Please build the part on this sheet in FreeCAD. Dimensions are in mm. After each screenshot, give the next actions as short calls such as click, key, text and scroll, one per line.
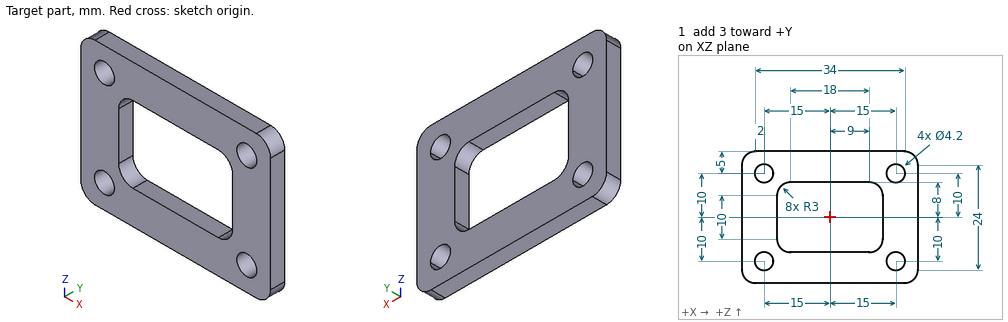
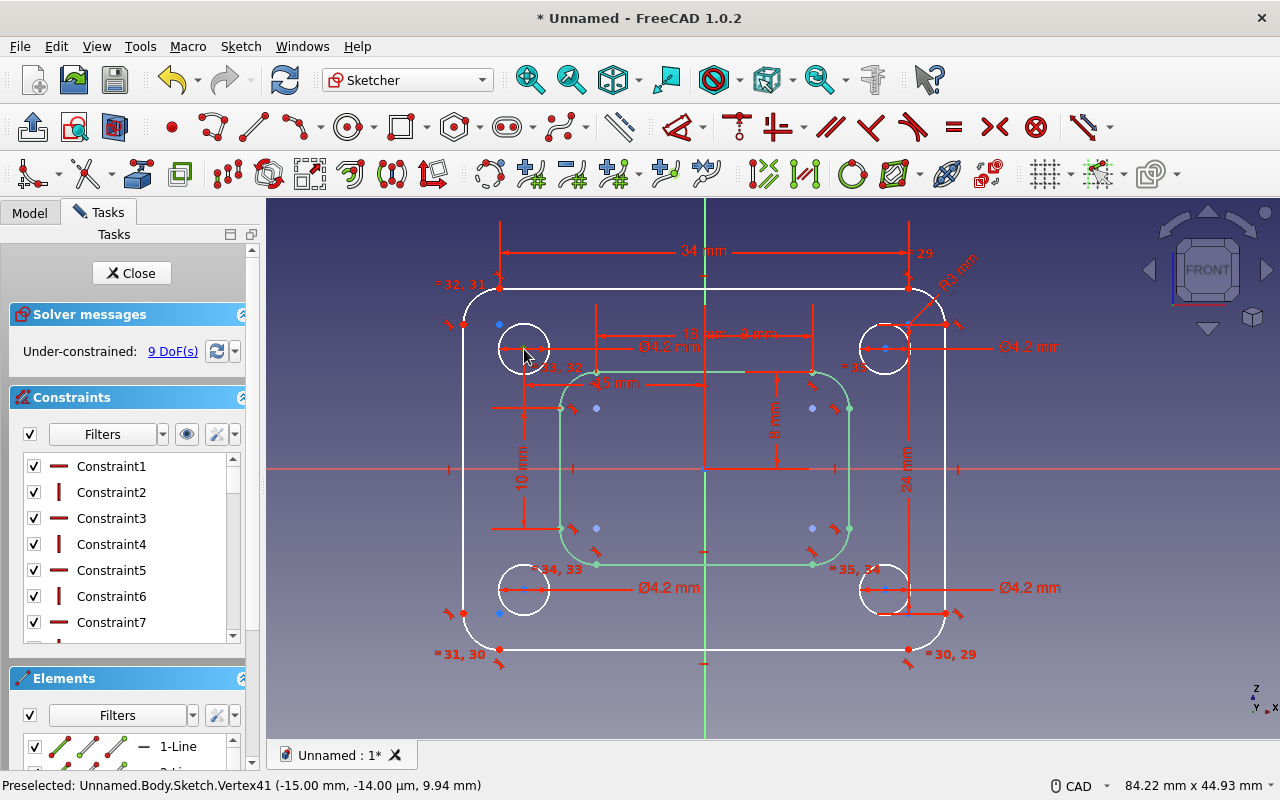
key(i)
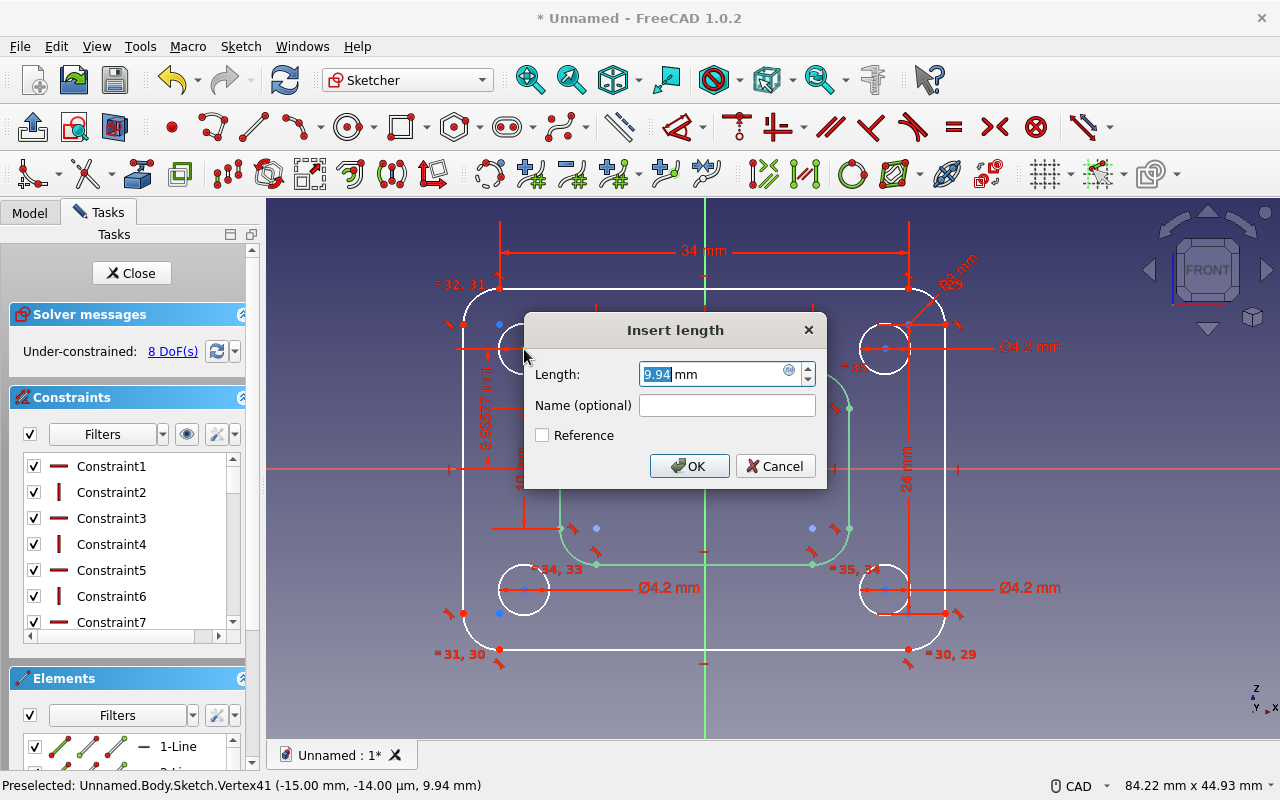
text(10)
key(Return)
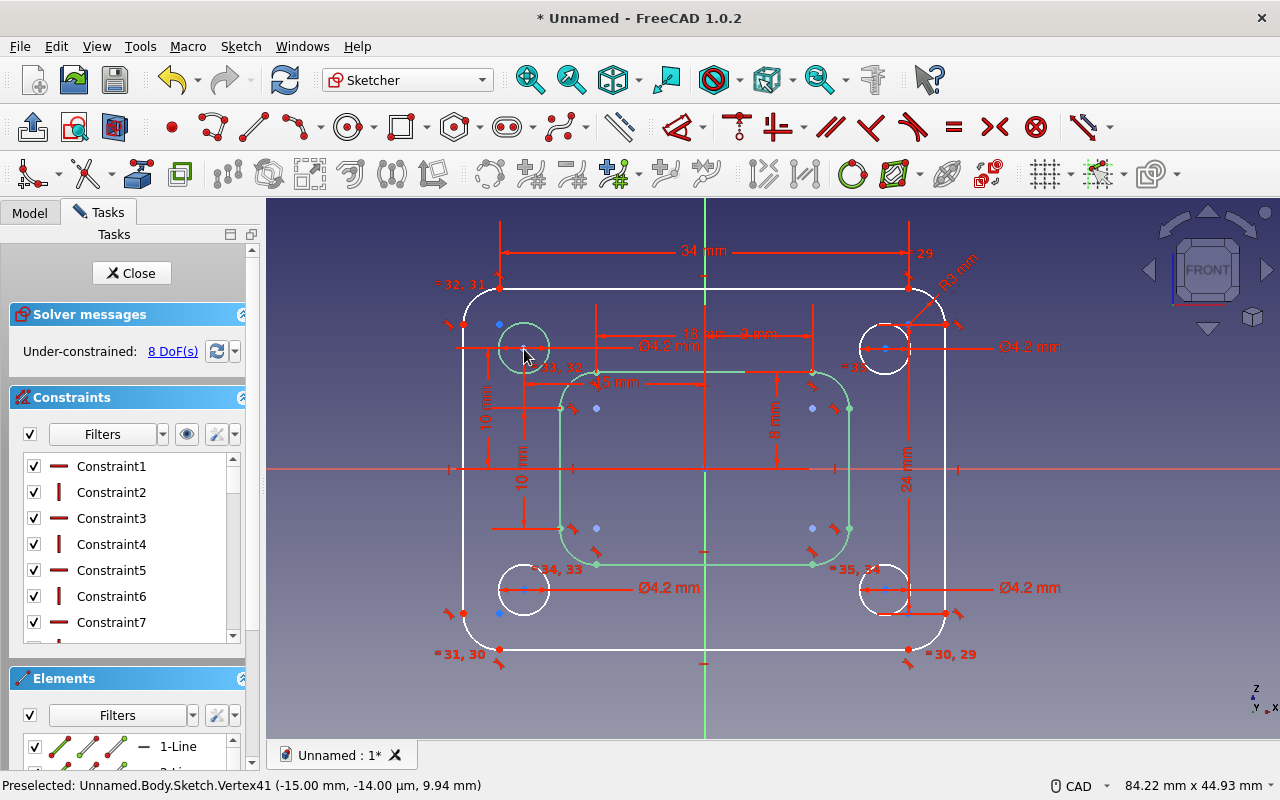
click(885, 349)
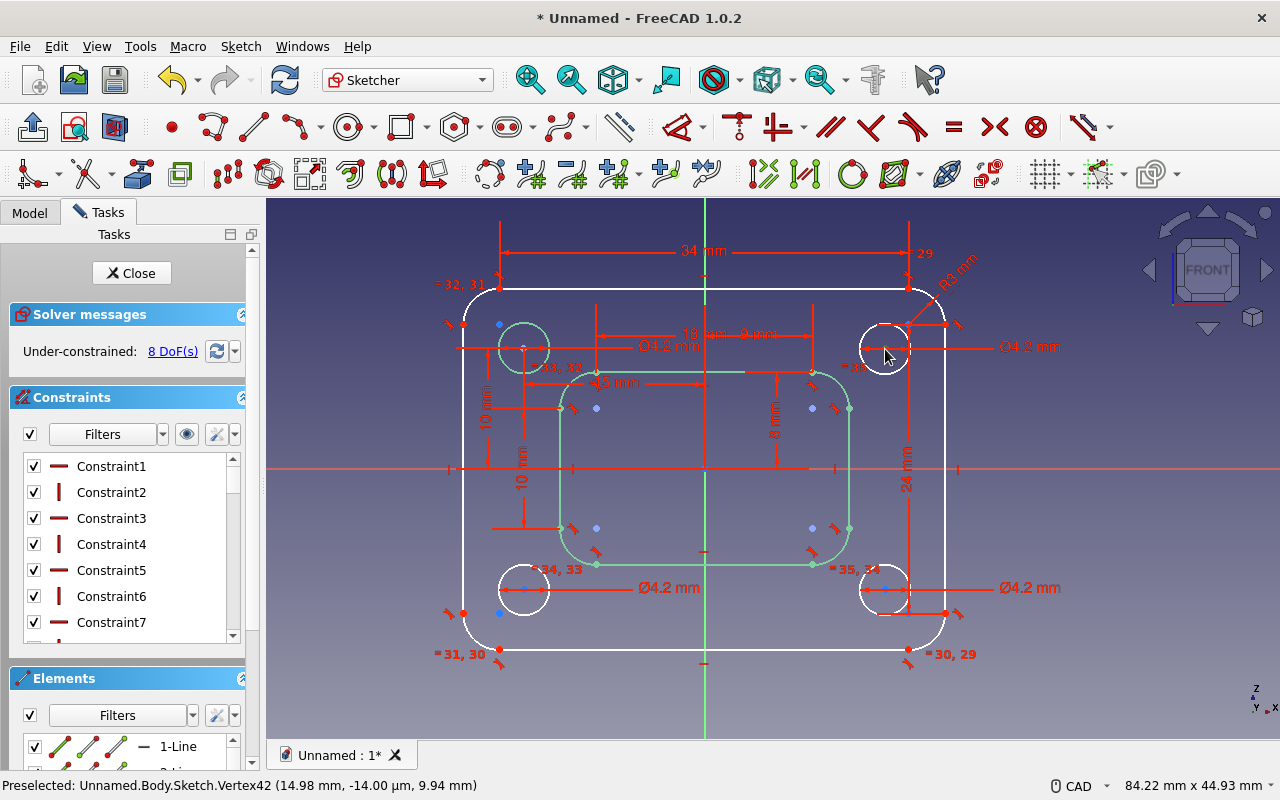
key(l)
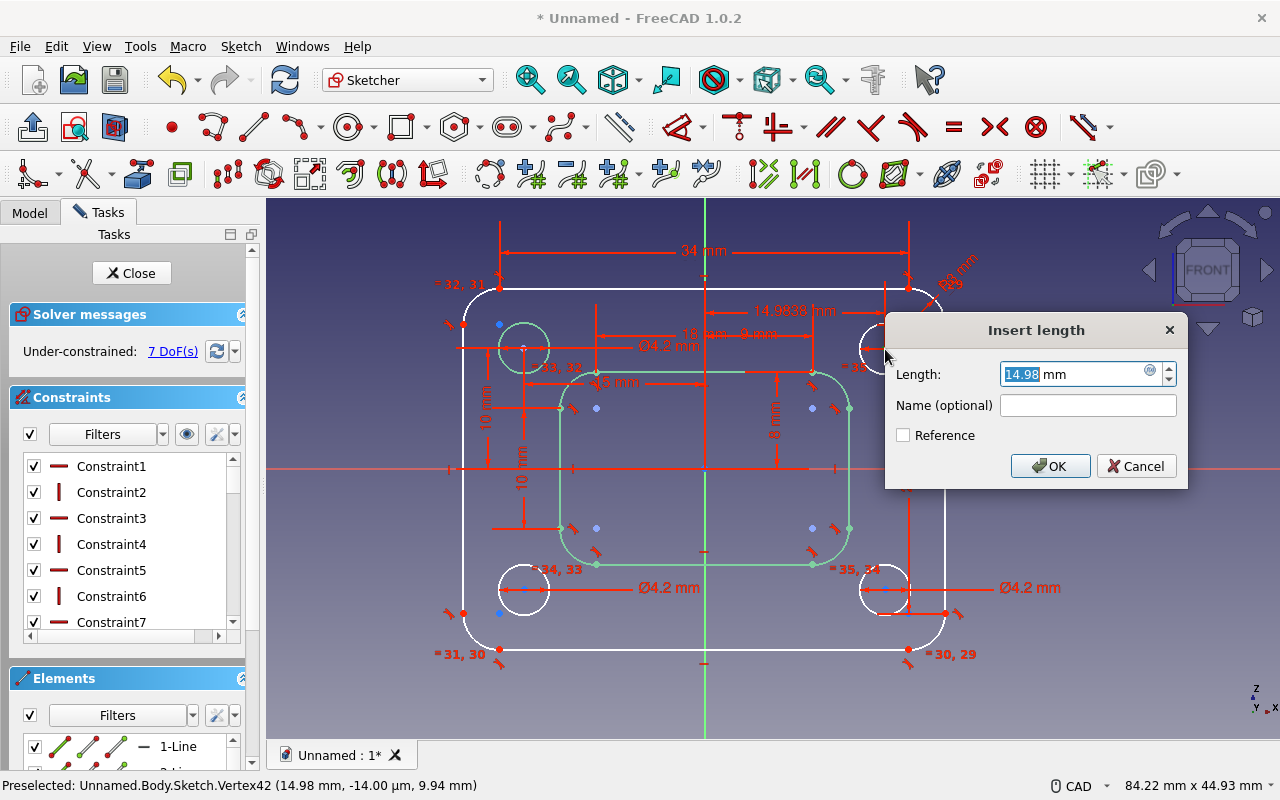
text(15)
key(Return)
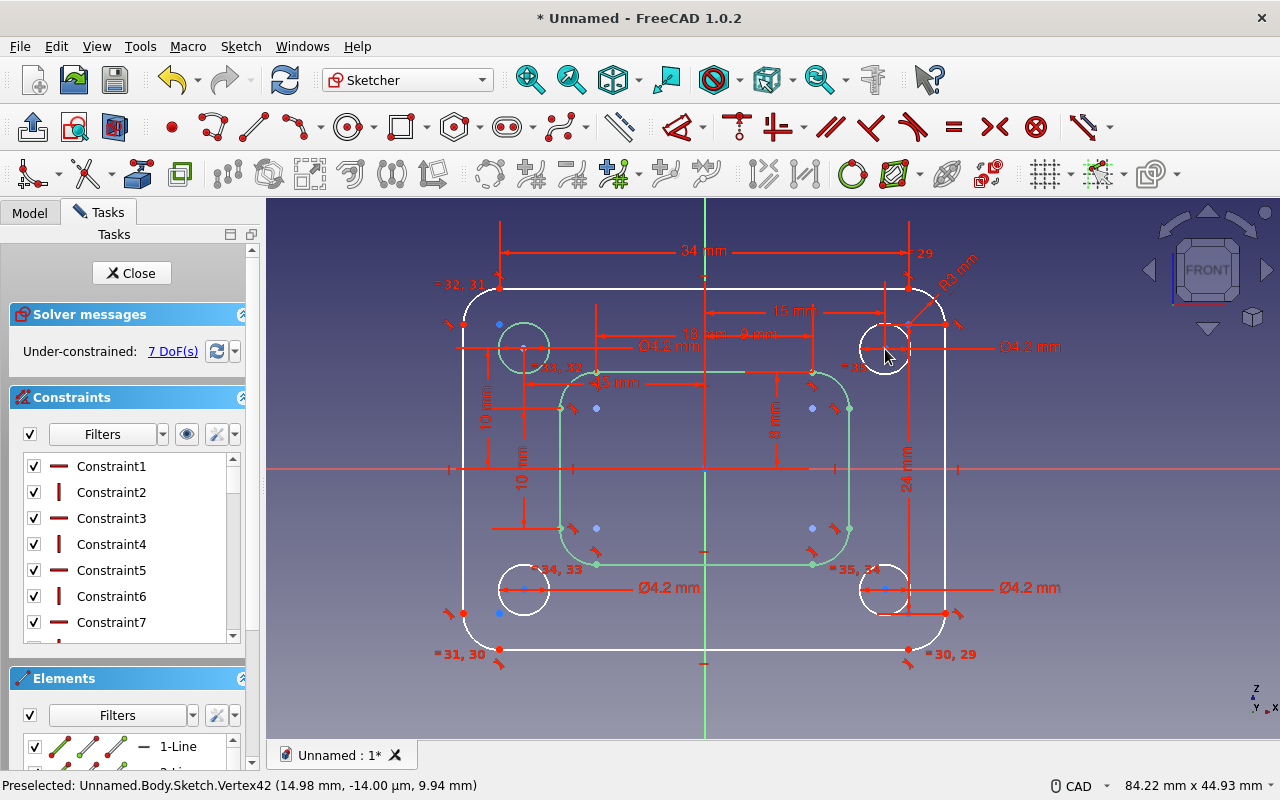
click(885, 349)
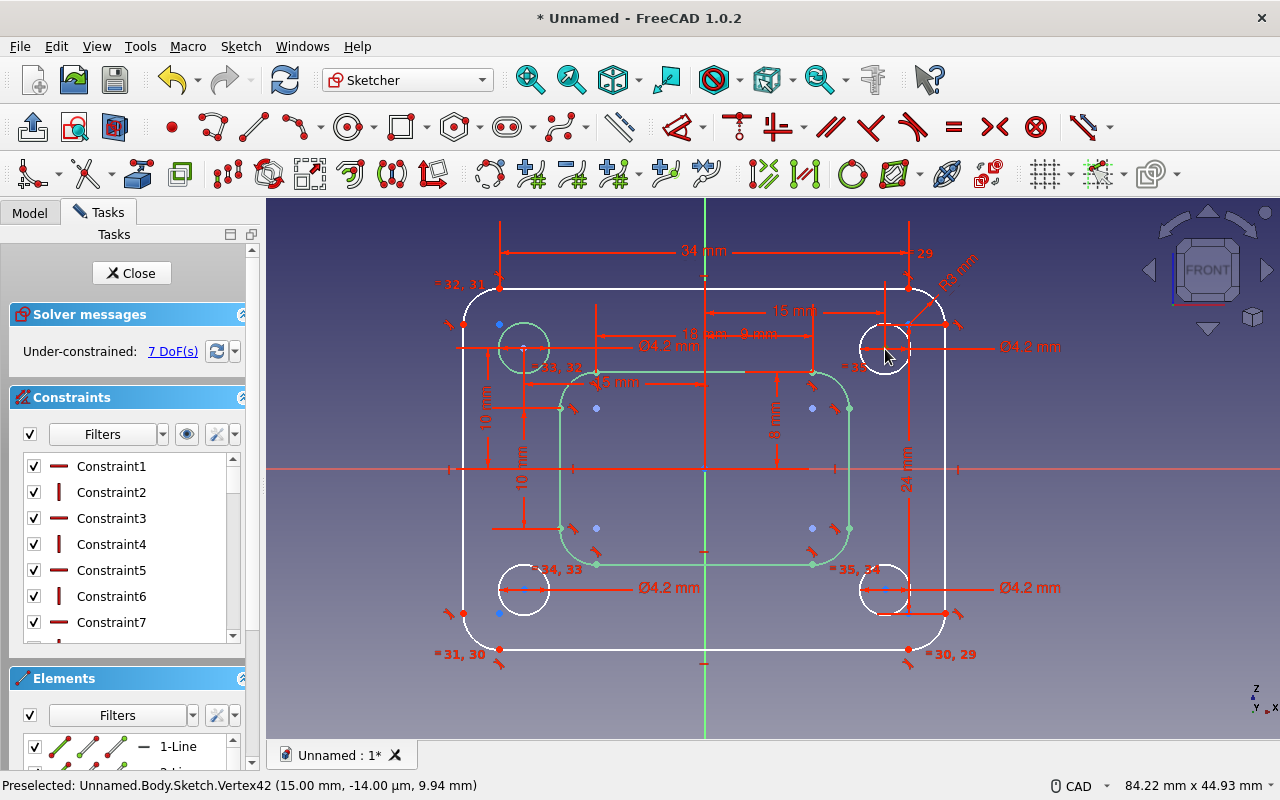
key(i)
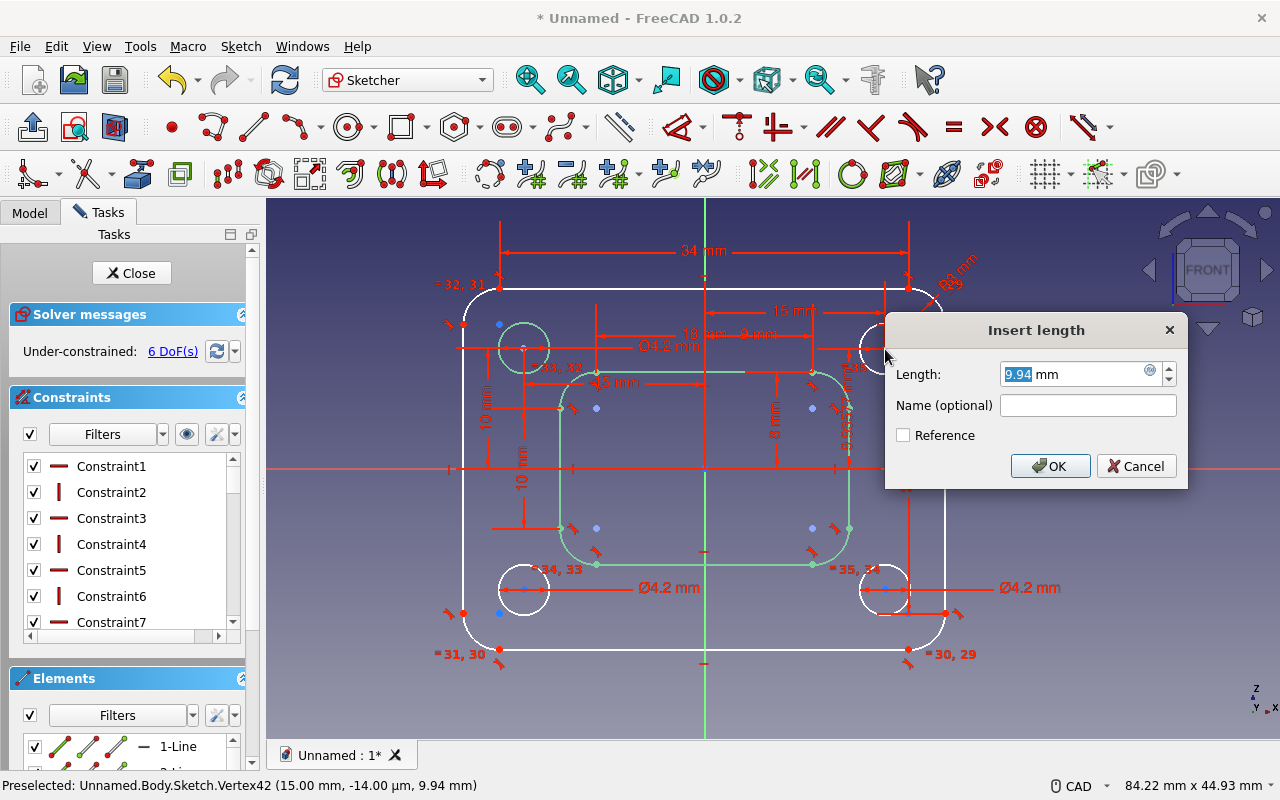
text(10)
key(Return)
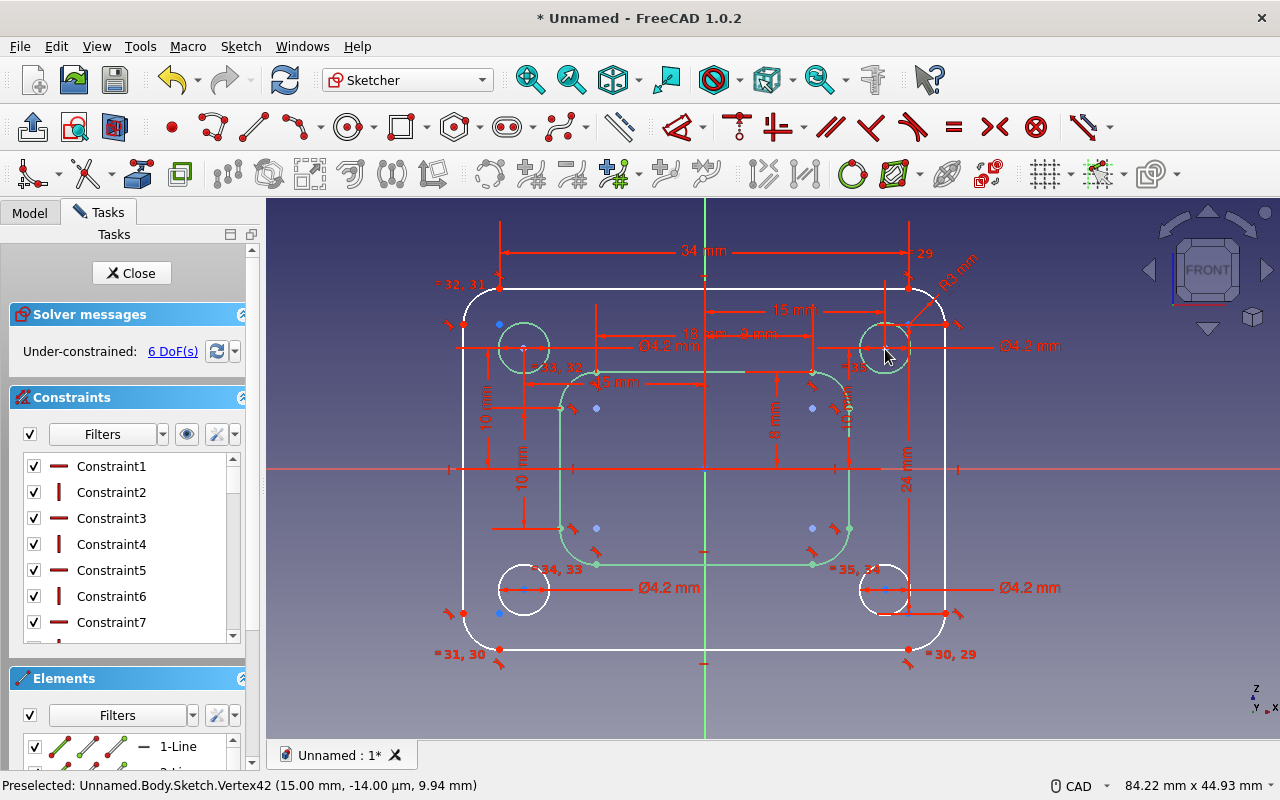
click(524, 590)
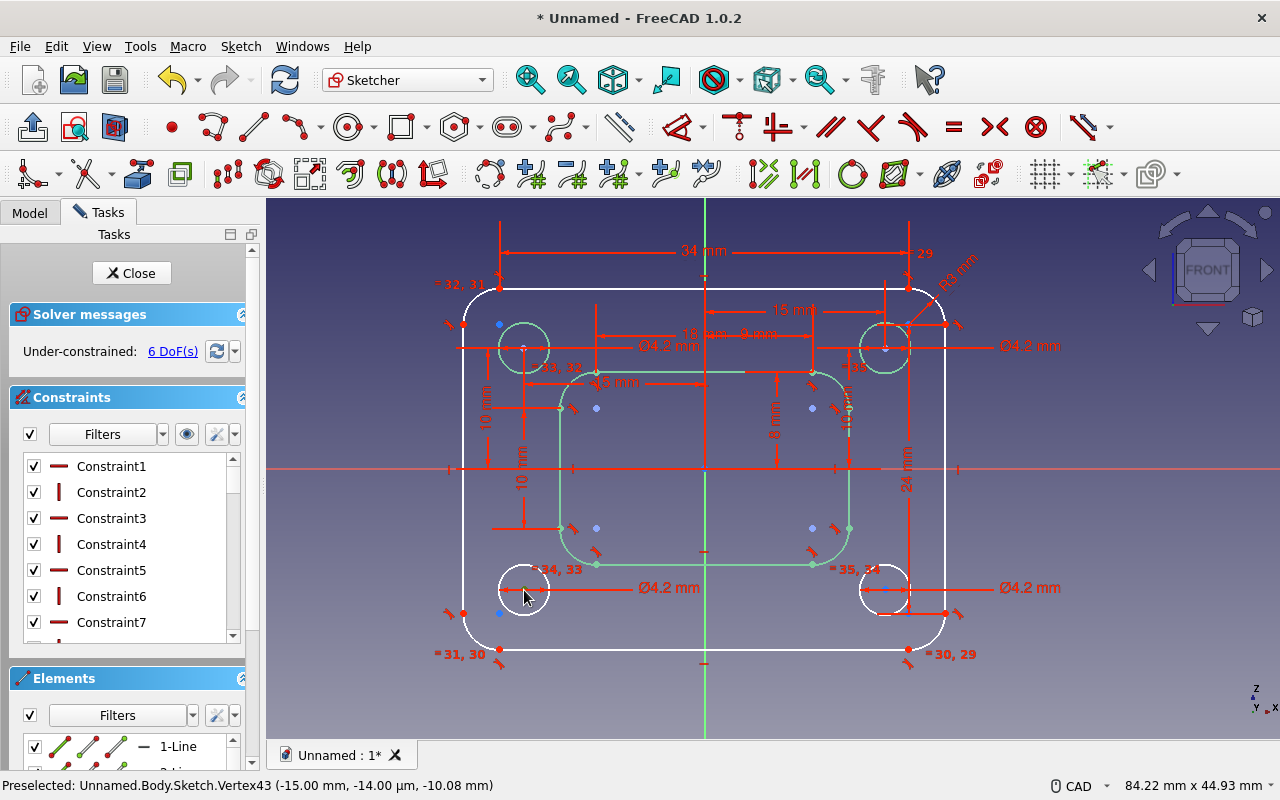
key(l)